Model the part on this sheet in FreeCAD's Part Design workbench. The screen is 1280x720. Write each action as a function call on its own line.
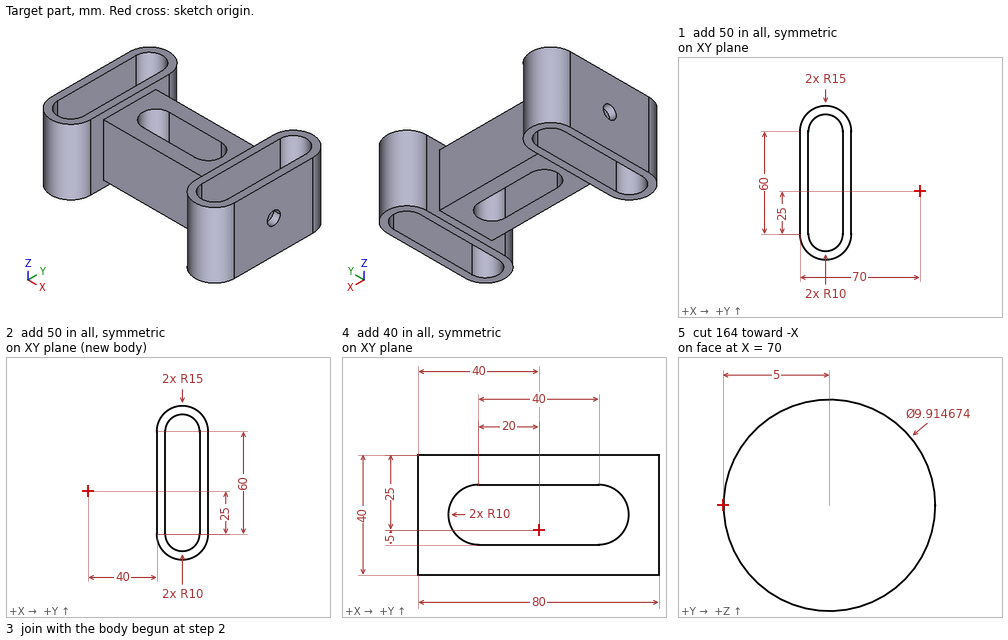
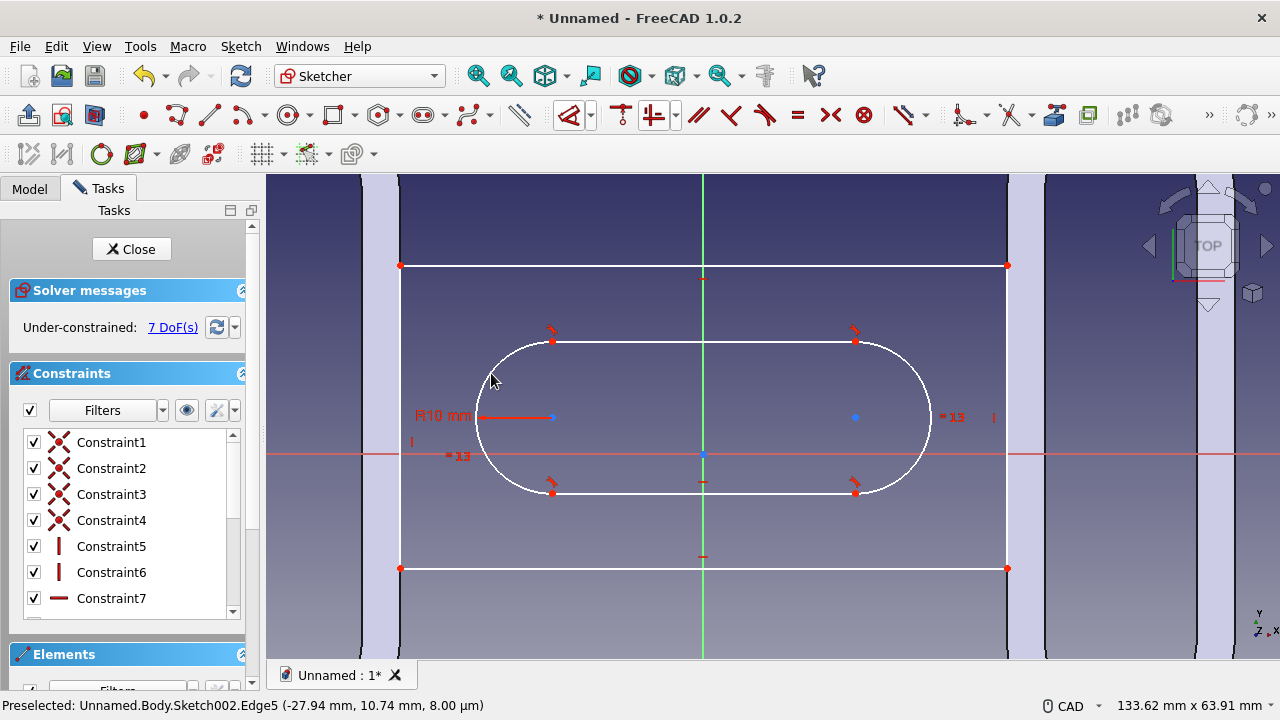
click(400, 357)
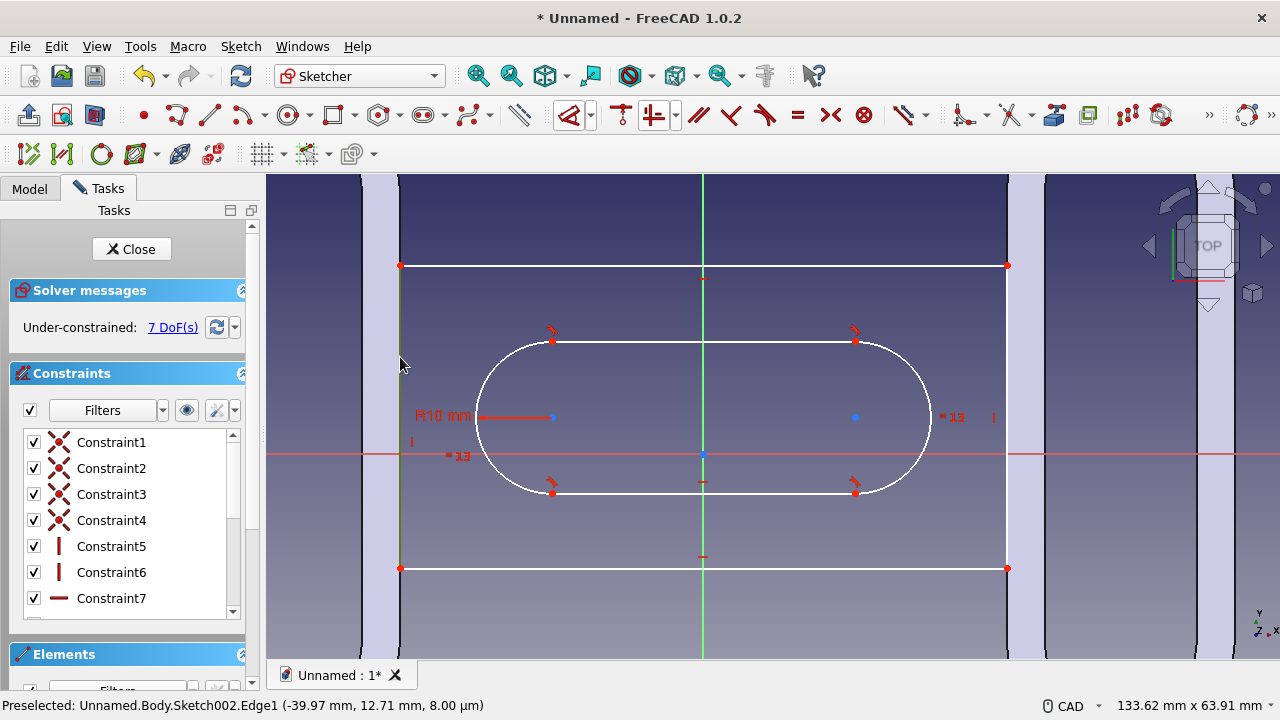
click(590, 116)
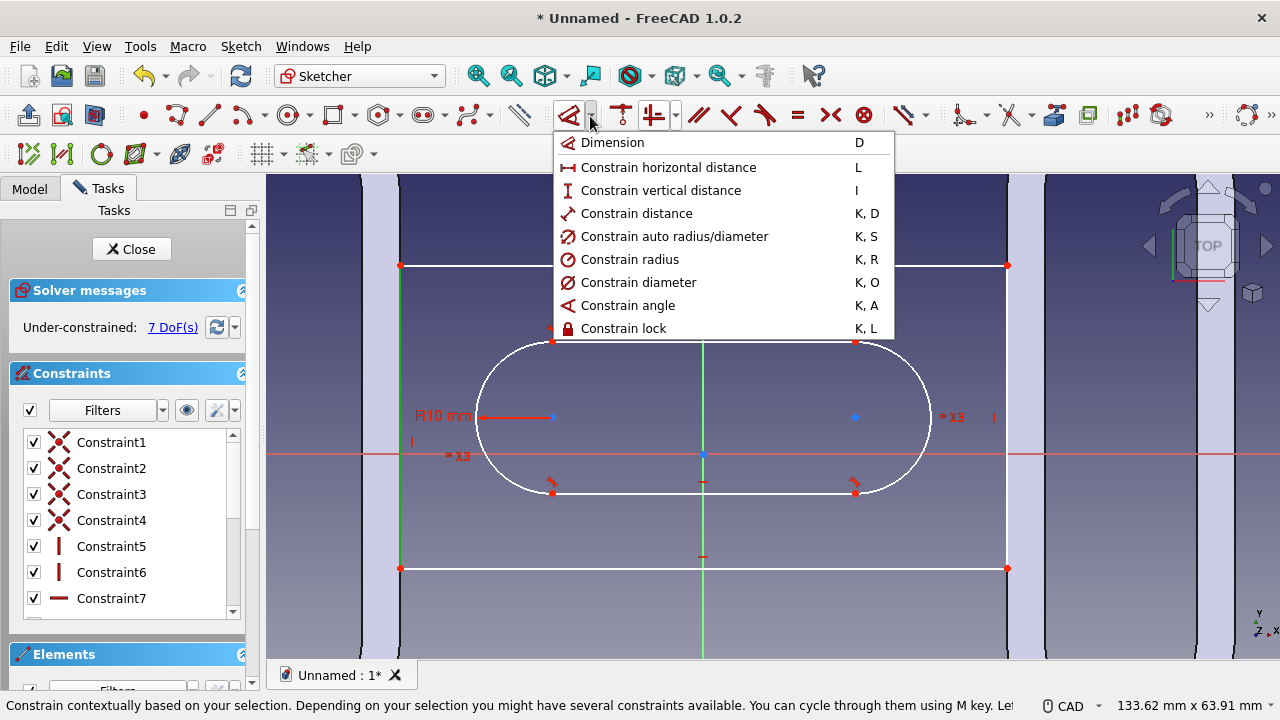
click(724, 190)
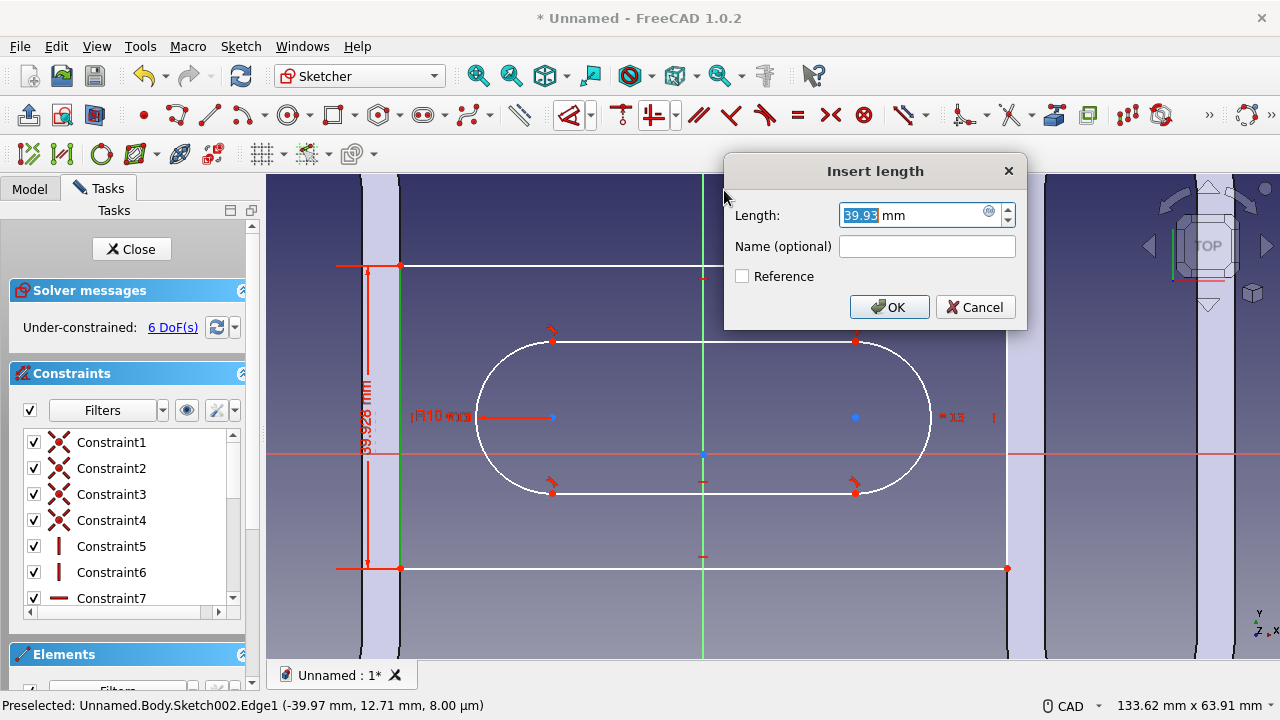
text(40)
key(Return)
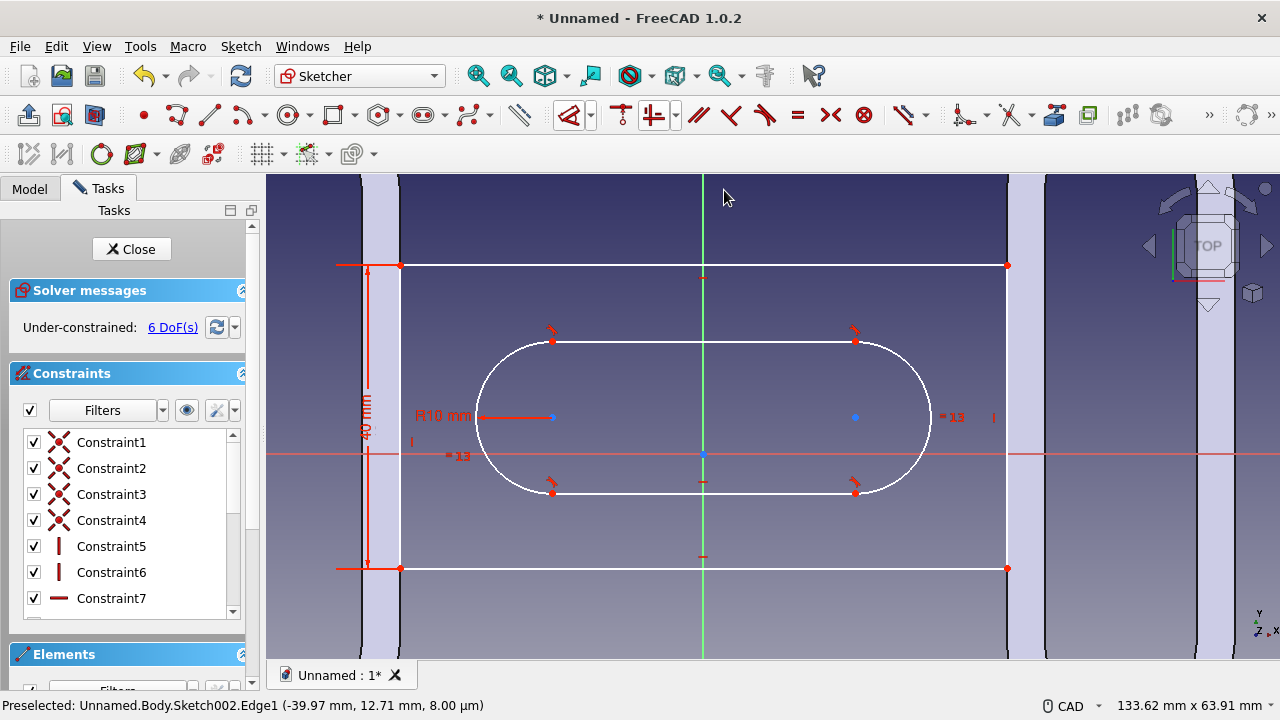
click(582, 569)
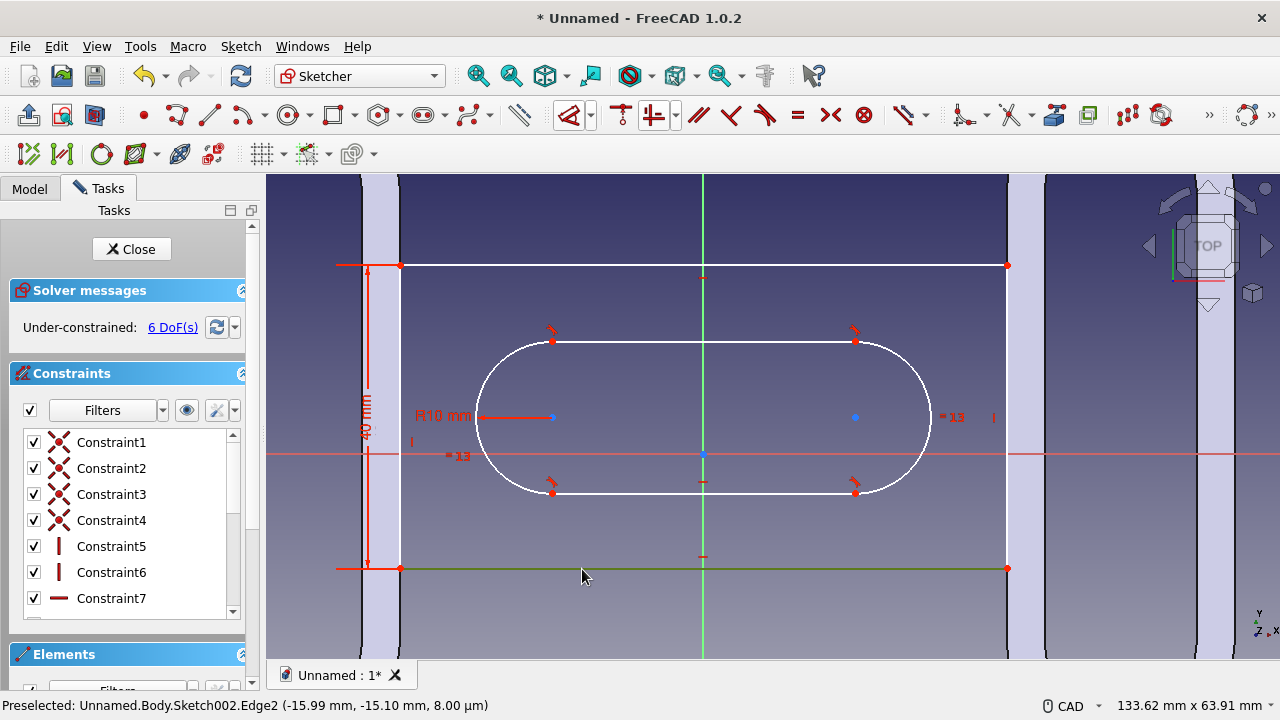
key(l)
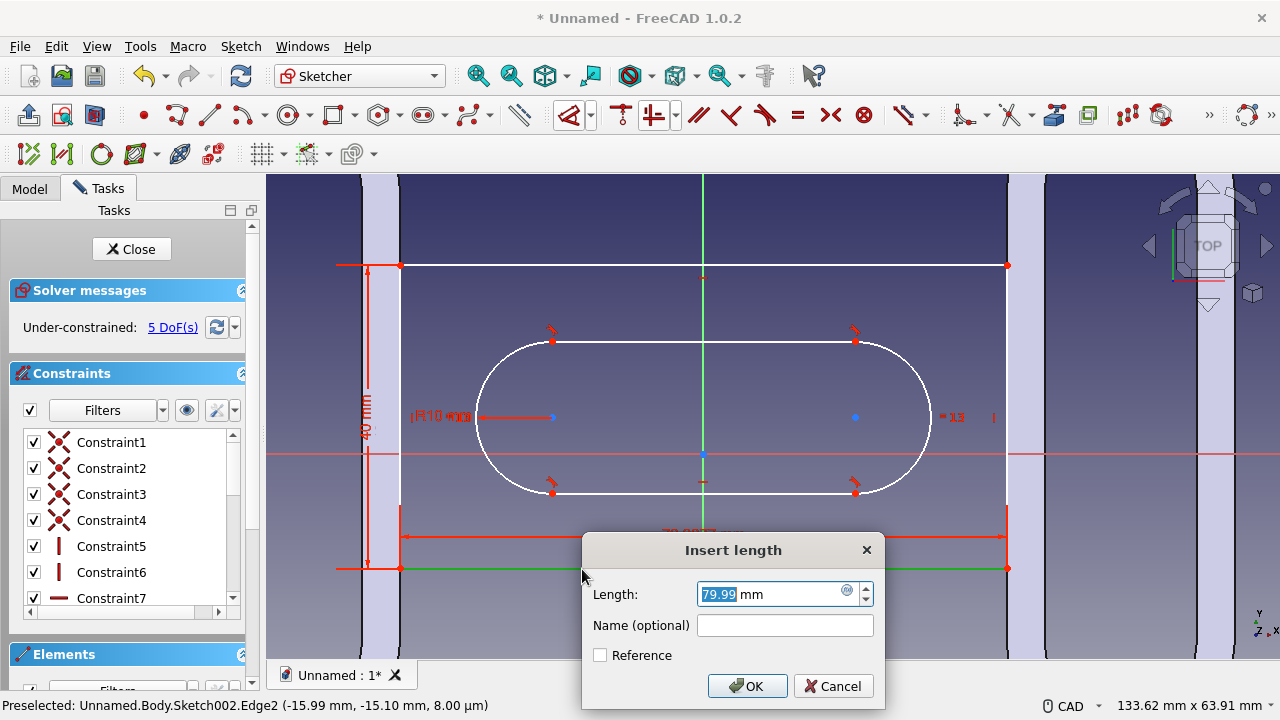
text(80)
key(Return)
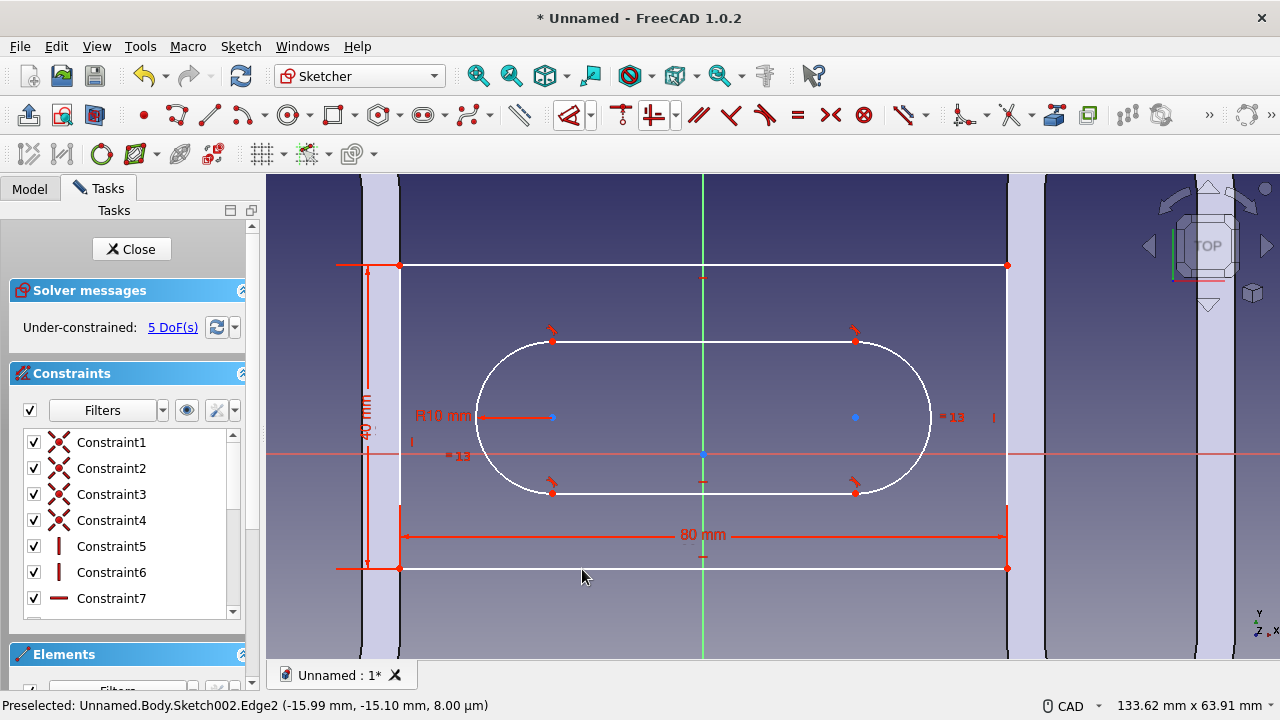
click(643, 342)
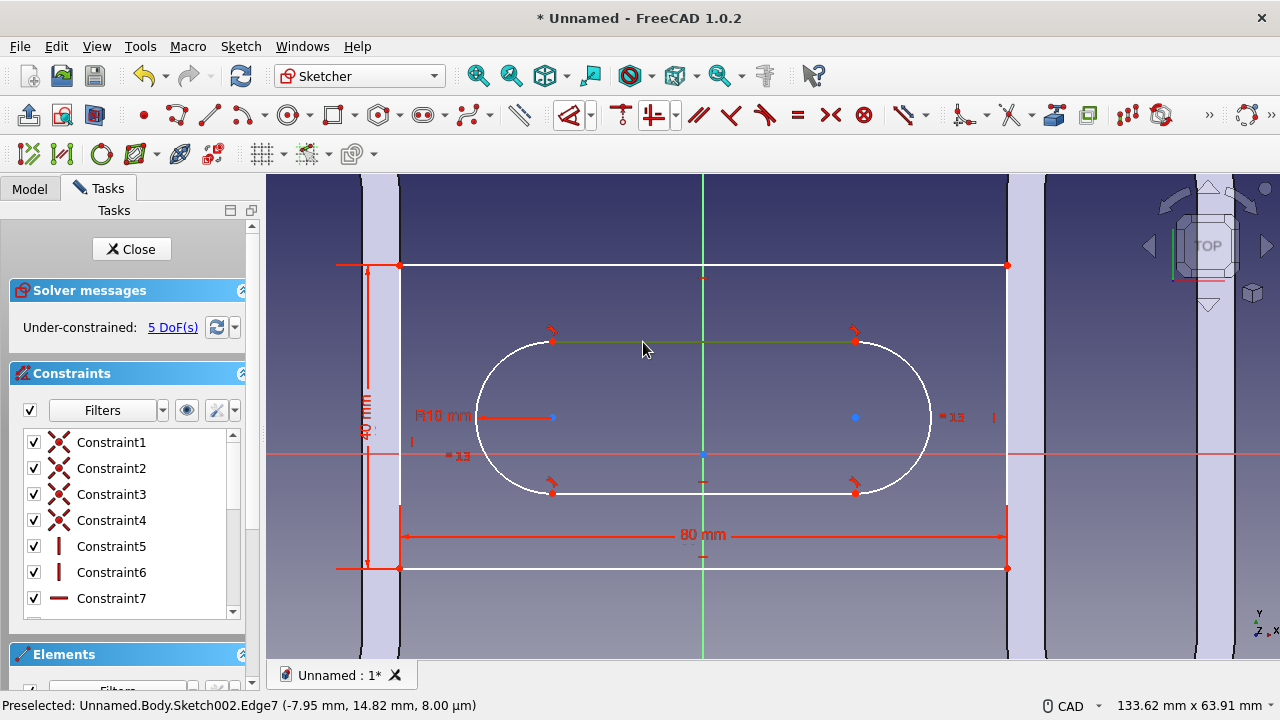
click(590, 116)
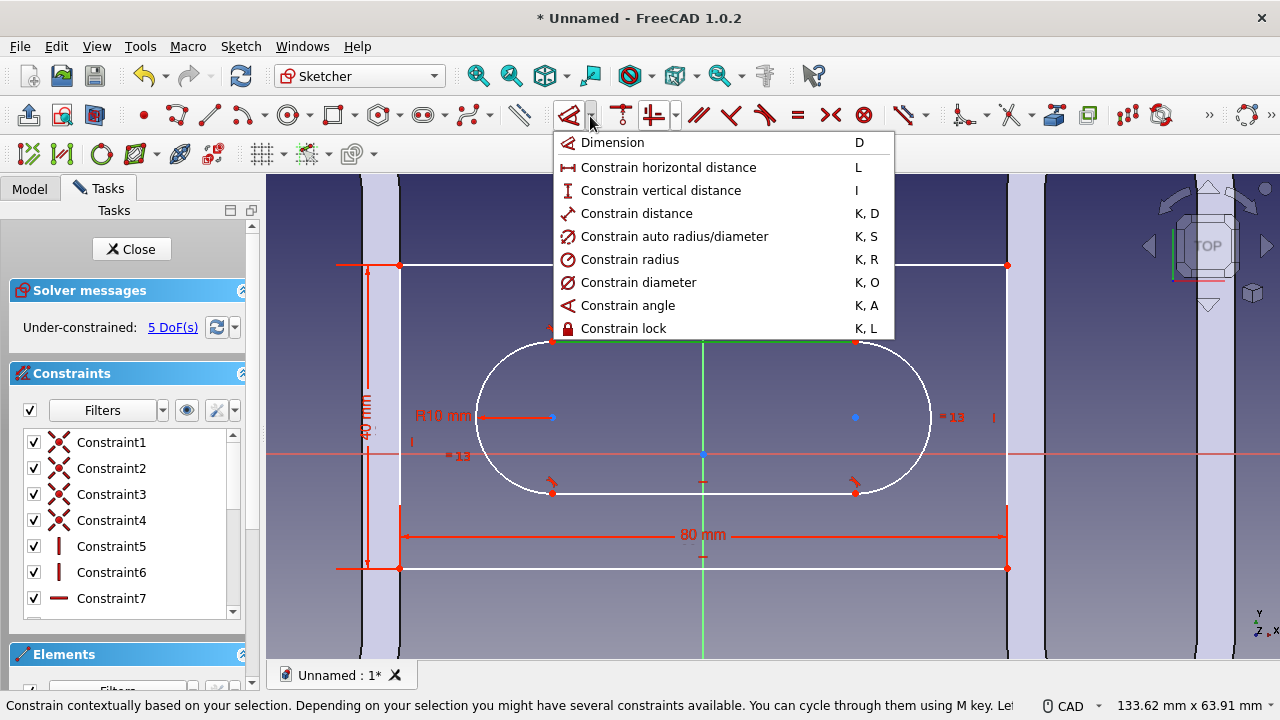
click(724, 168)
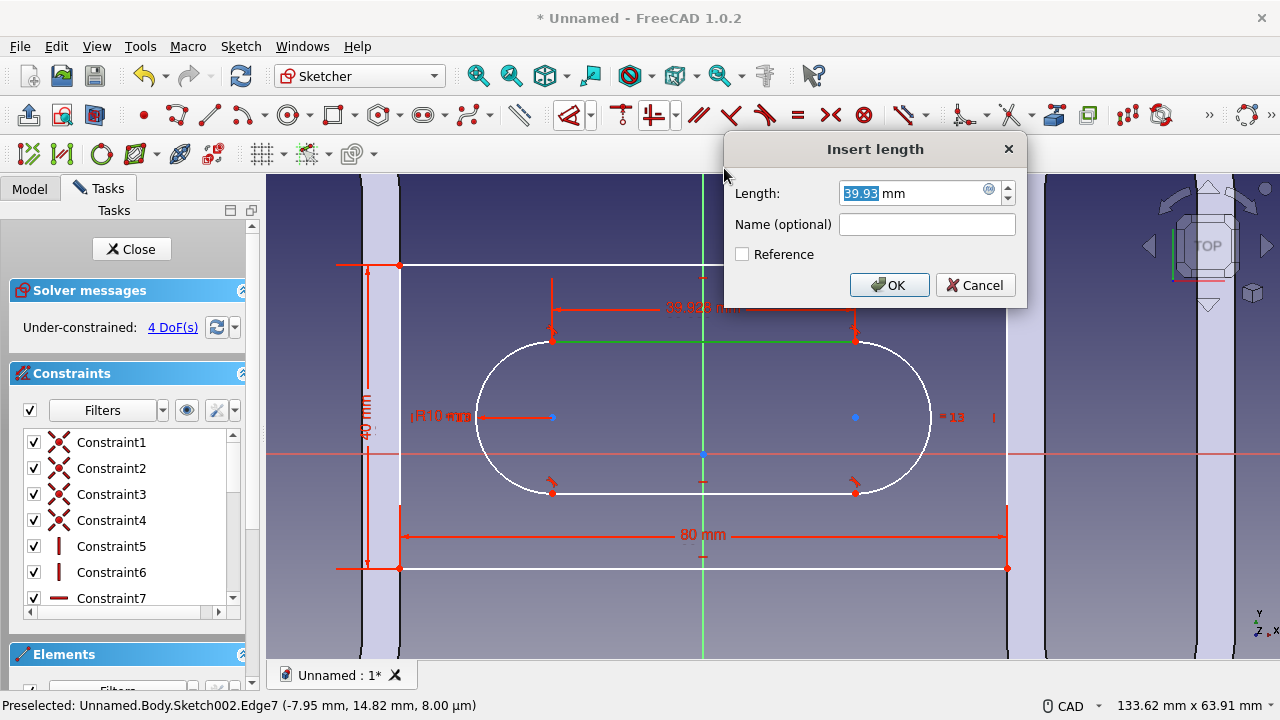
text(40)
key(Return)